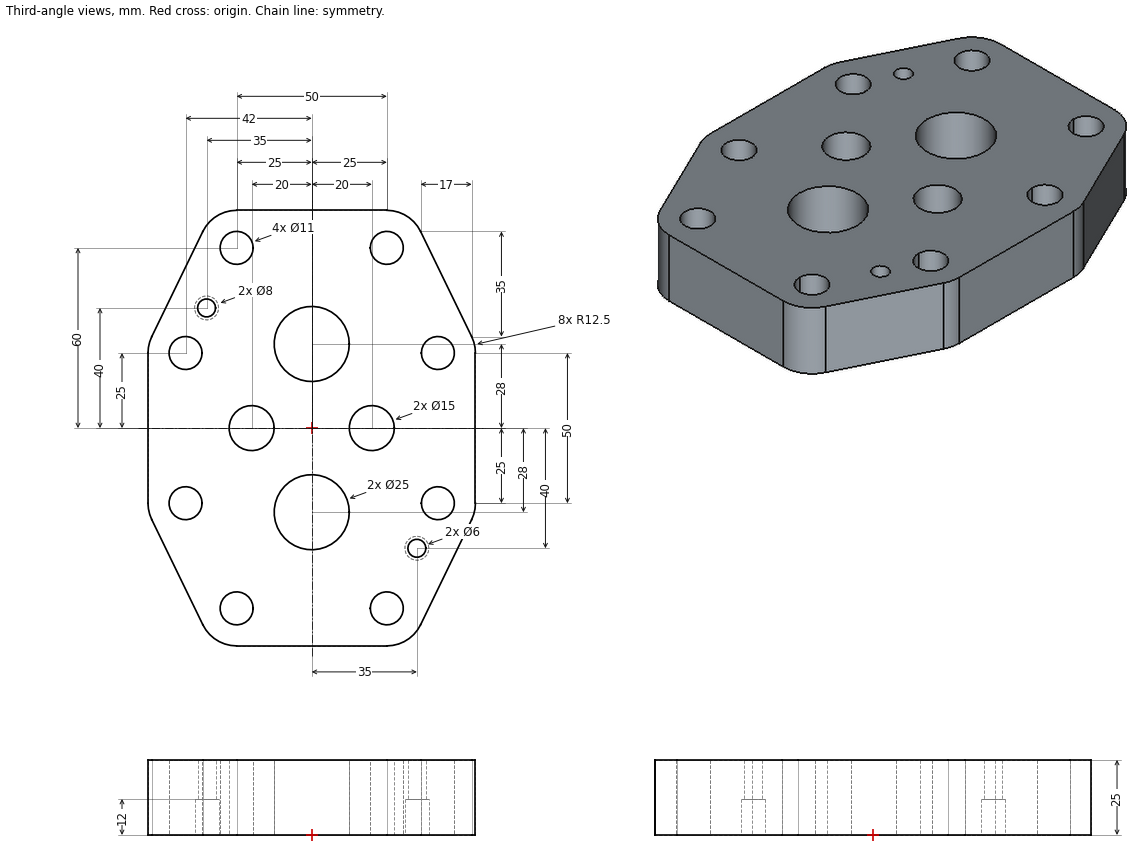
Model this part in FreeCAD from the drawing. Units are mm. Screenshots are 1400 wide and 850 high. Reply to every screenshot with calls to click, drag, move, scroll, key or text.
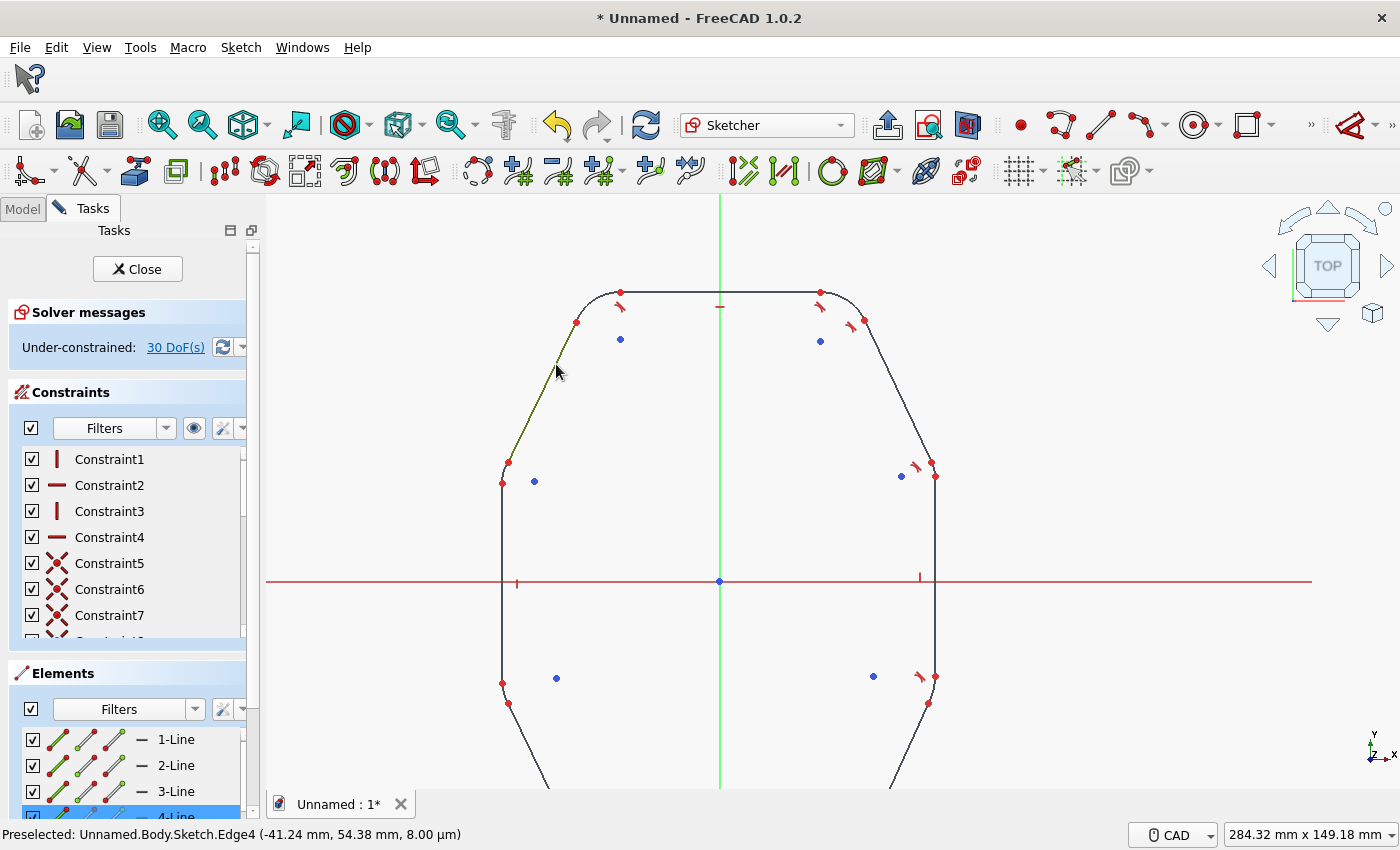
click(604, 295)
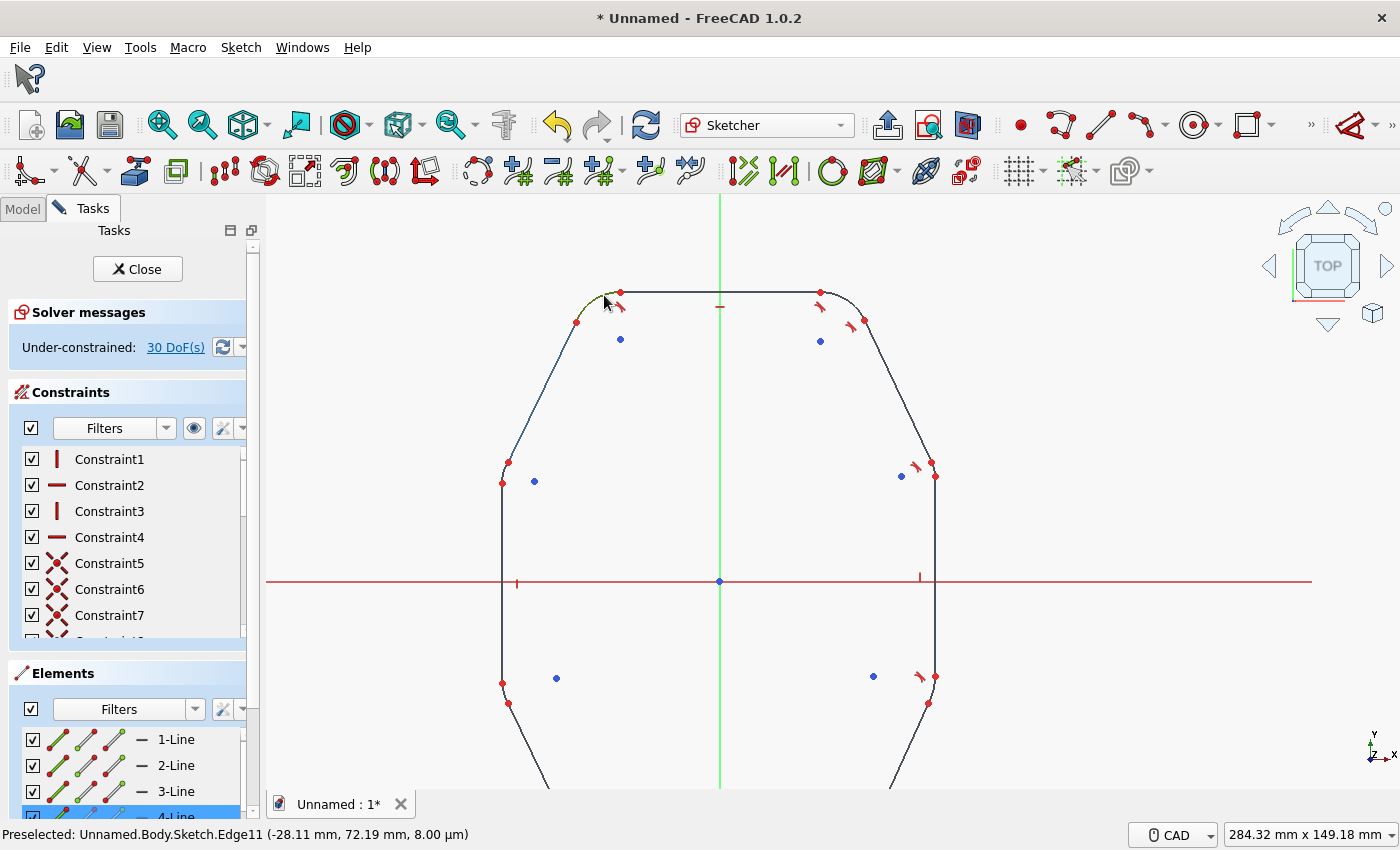
key(t)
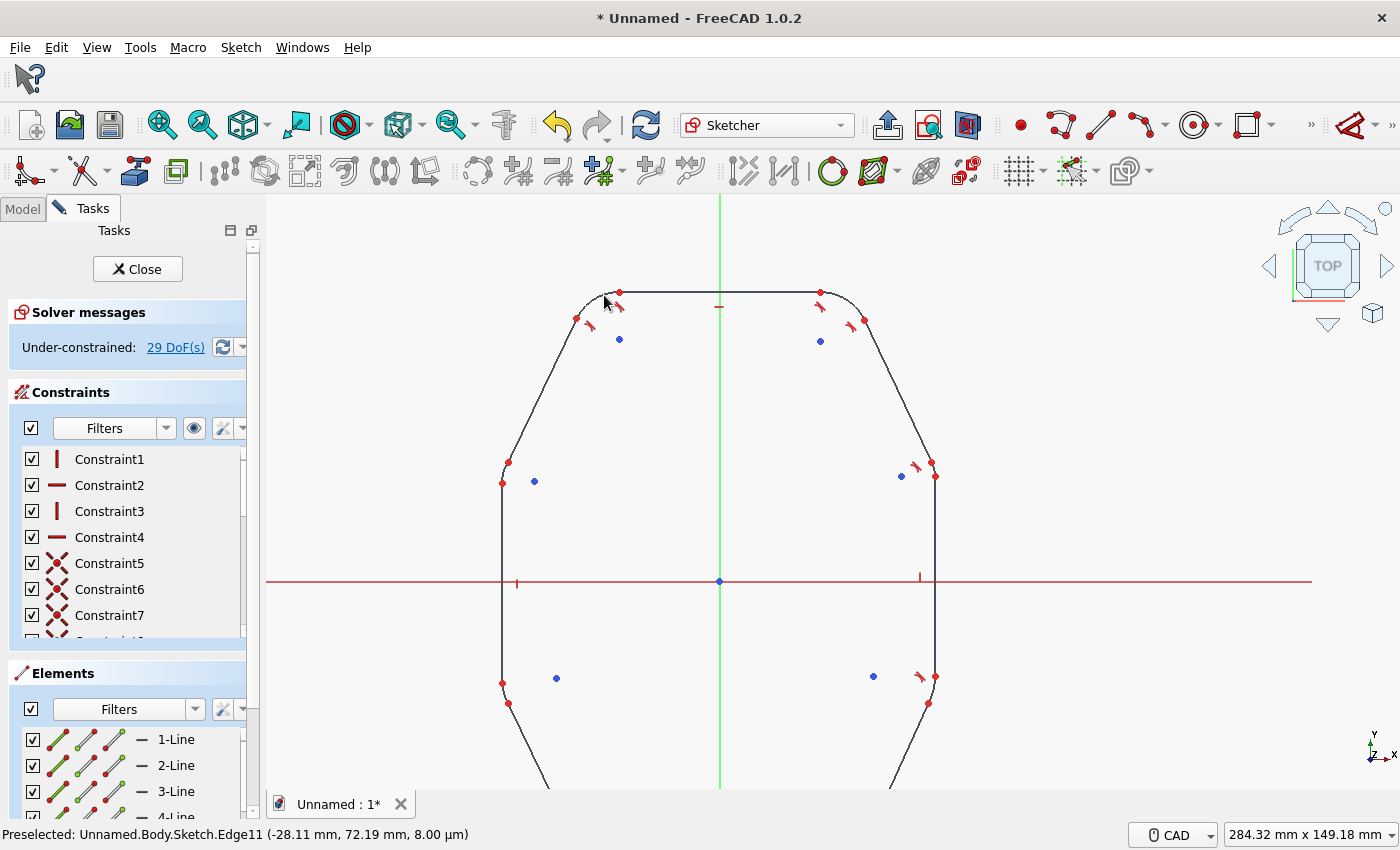
click(556, 362)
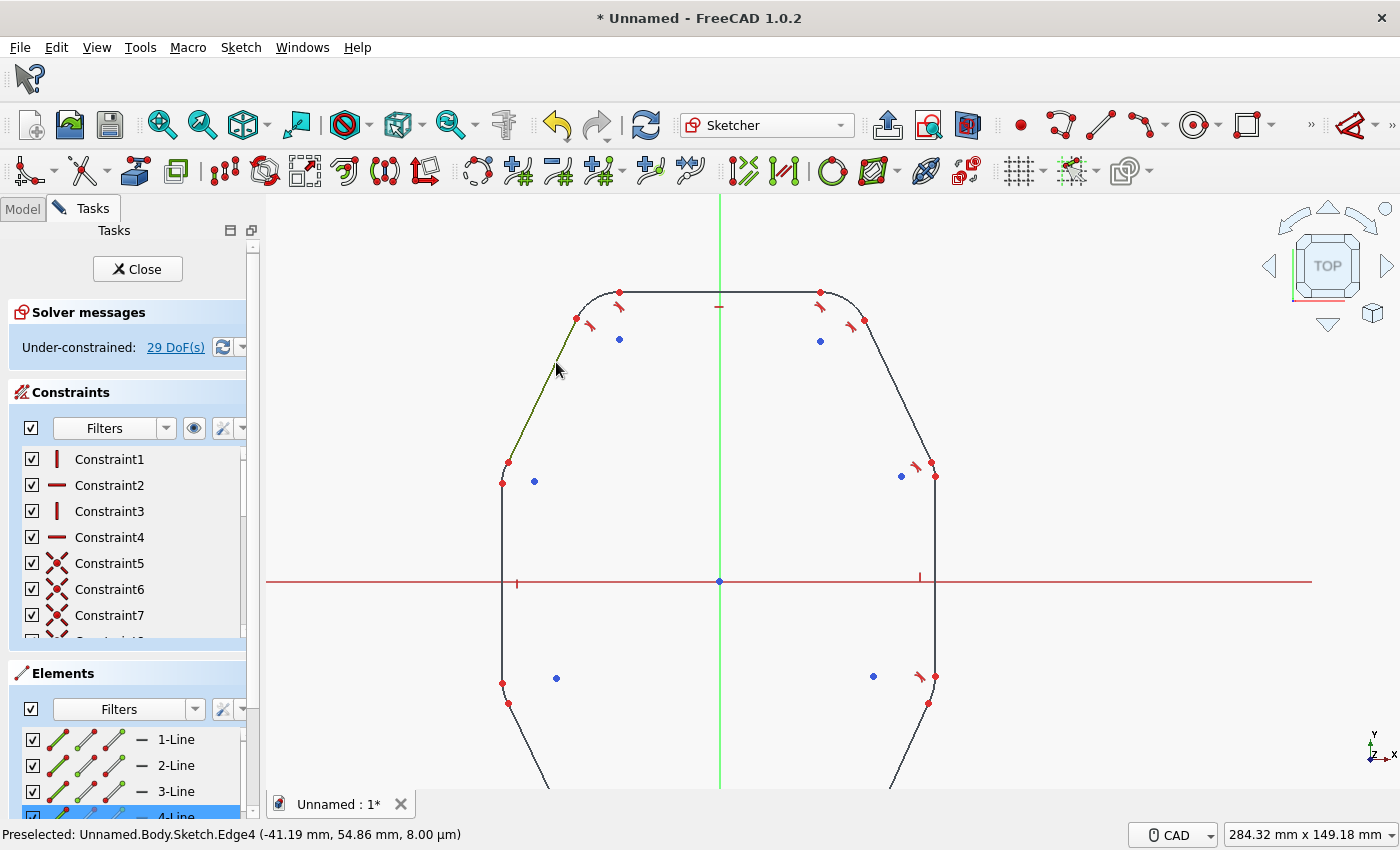
scroll(503, 472, up, 2)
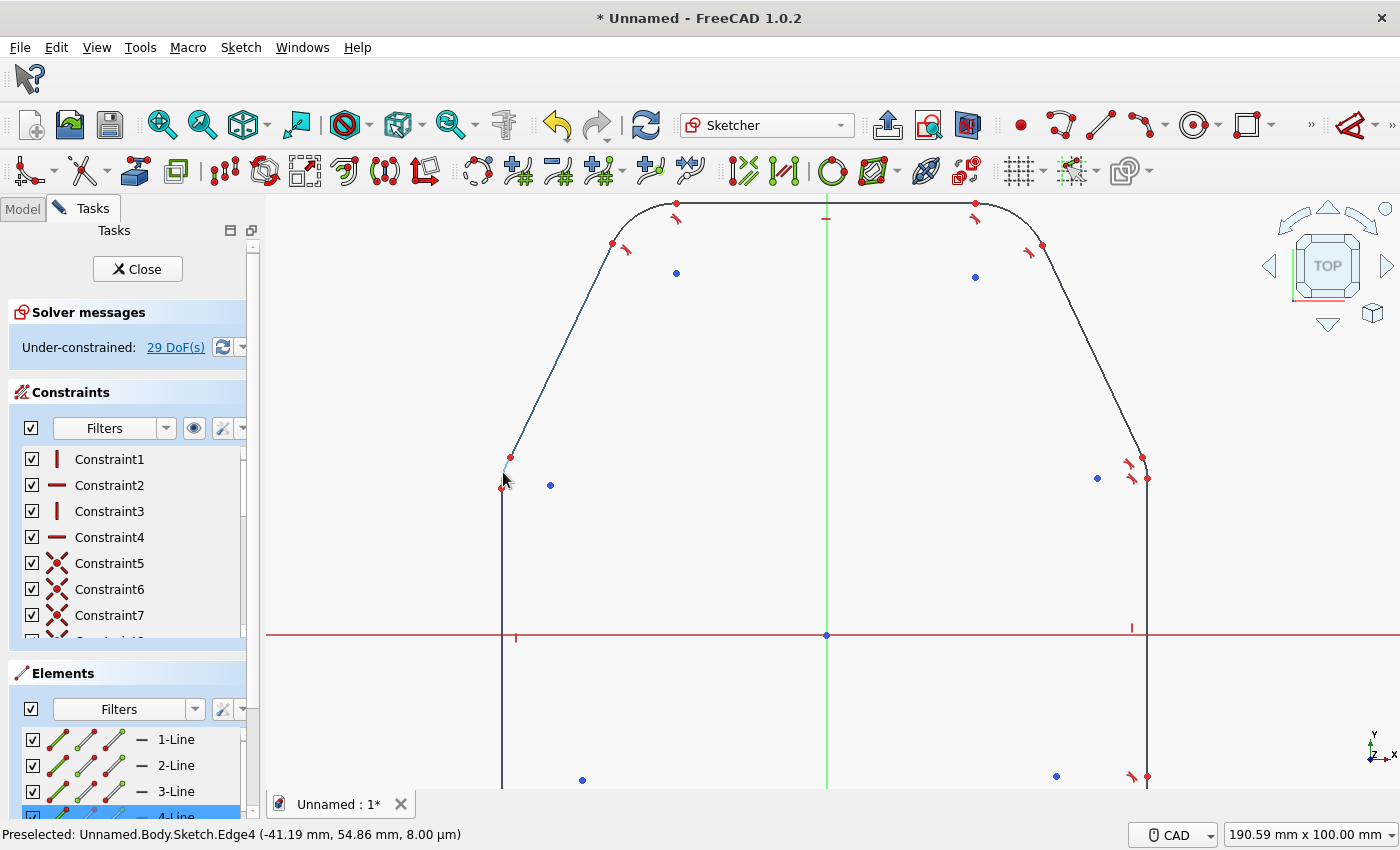
click(504, 472)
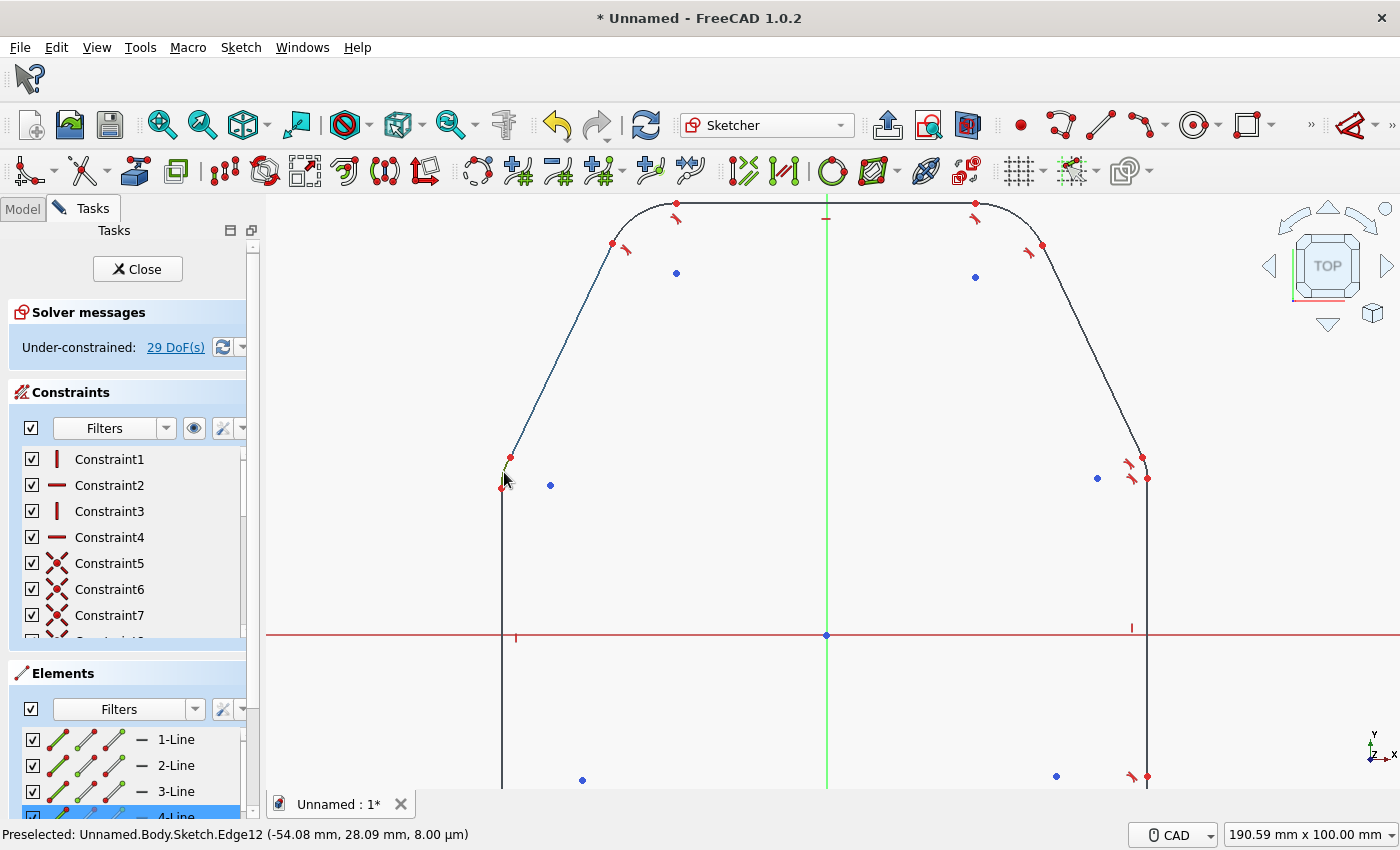
key(t)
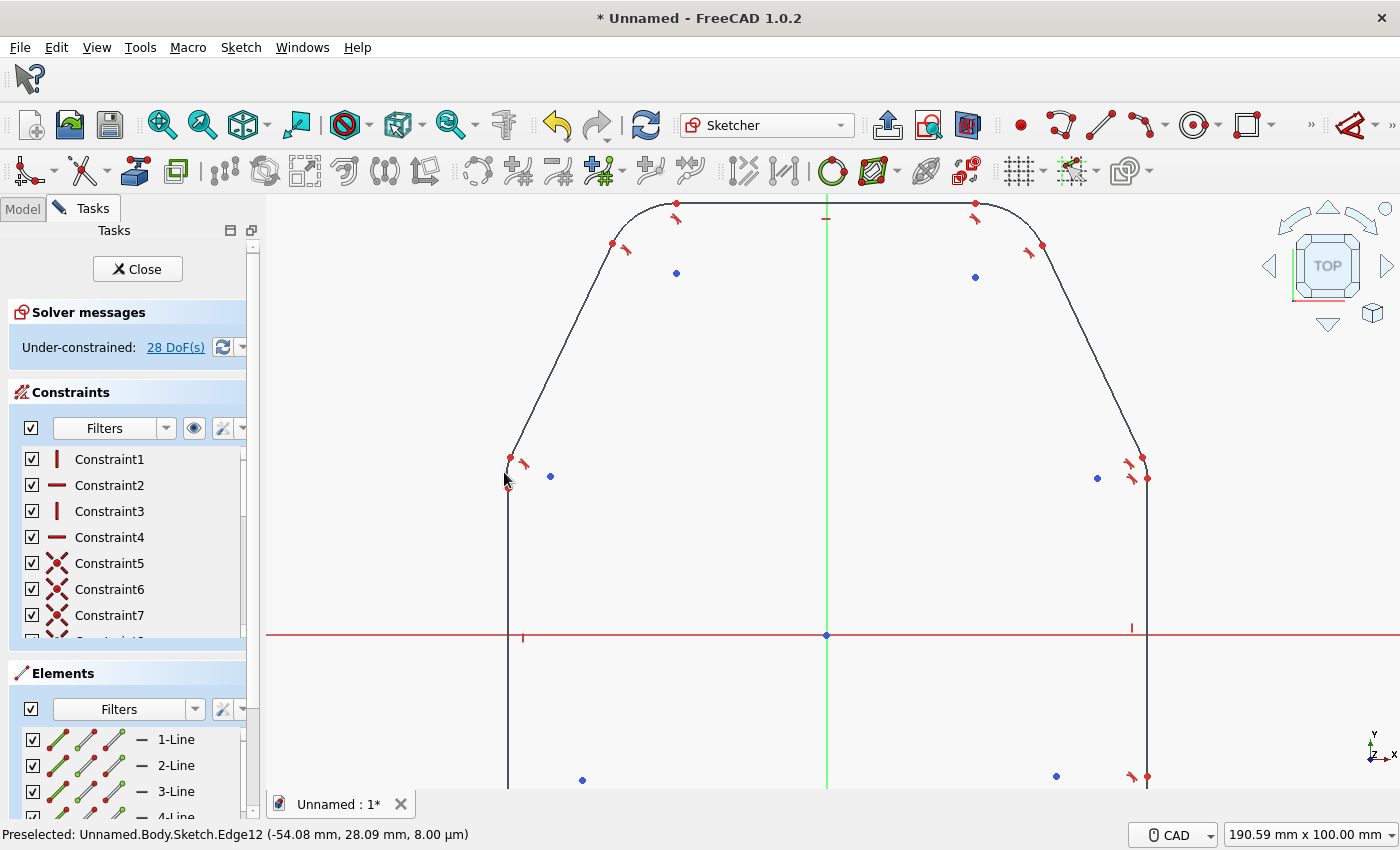
click(508, 578)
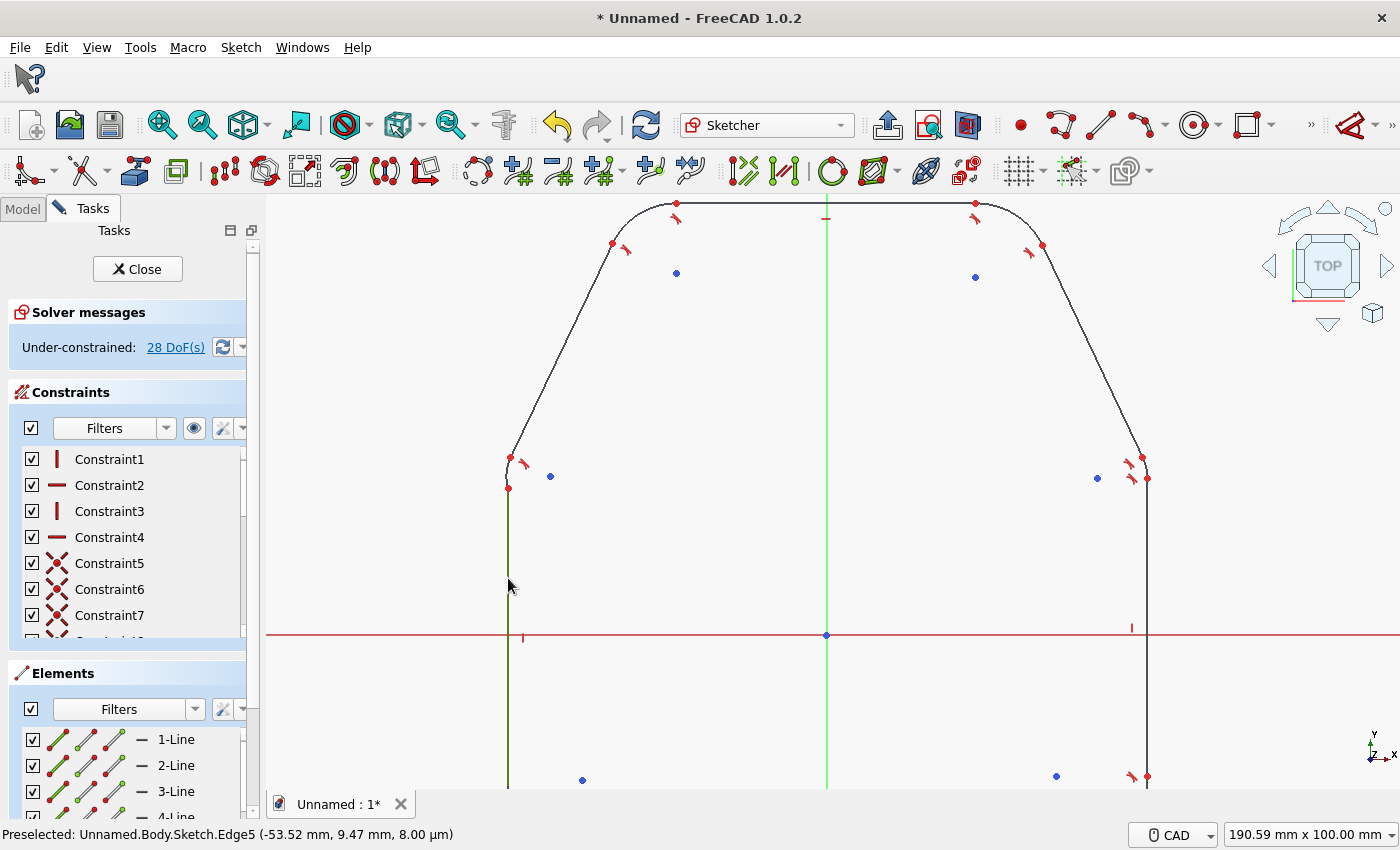
scroll(508, 466, up, 2)